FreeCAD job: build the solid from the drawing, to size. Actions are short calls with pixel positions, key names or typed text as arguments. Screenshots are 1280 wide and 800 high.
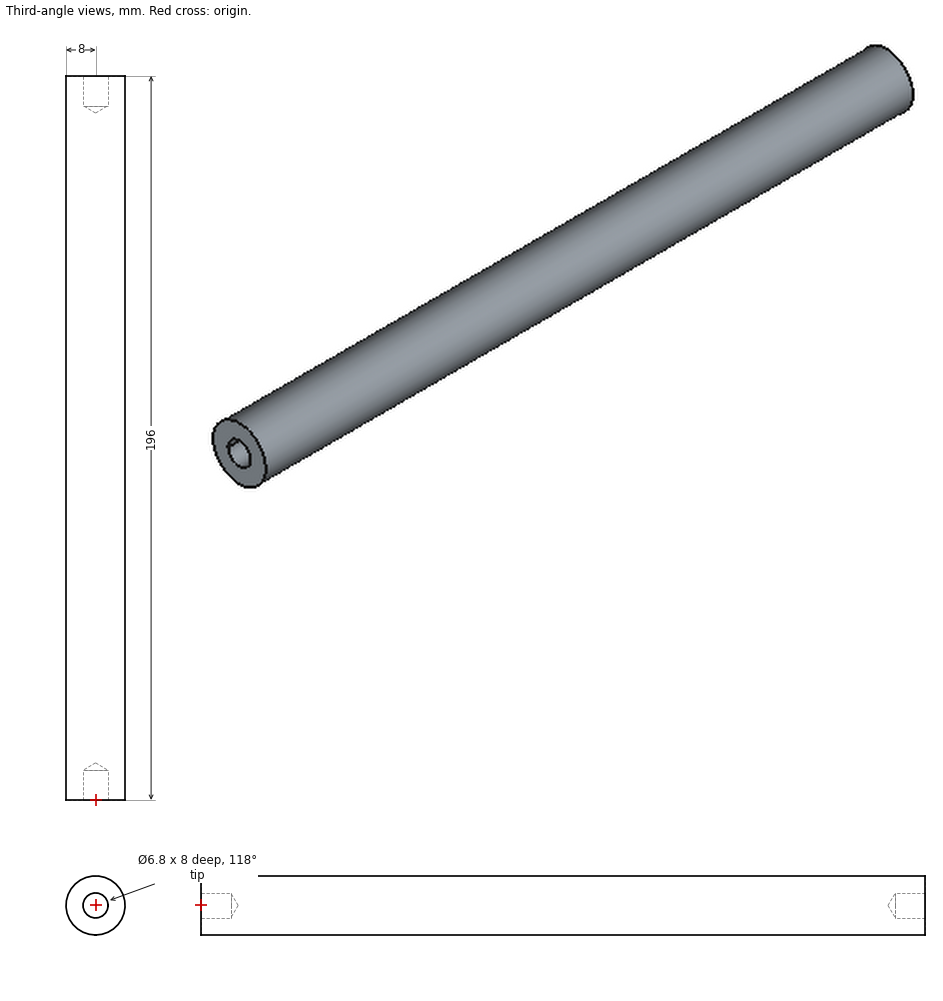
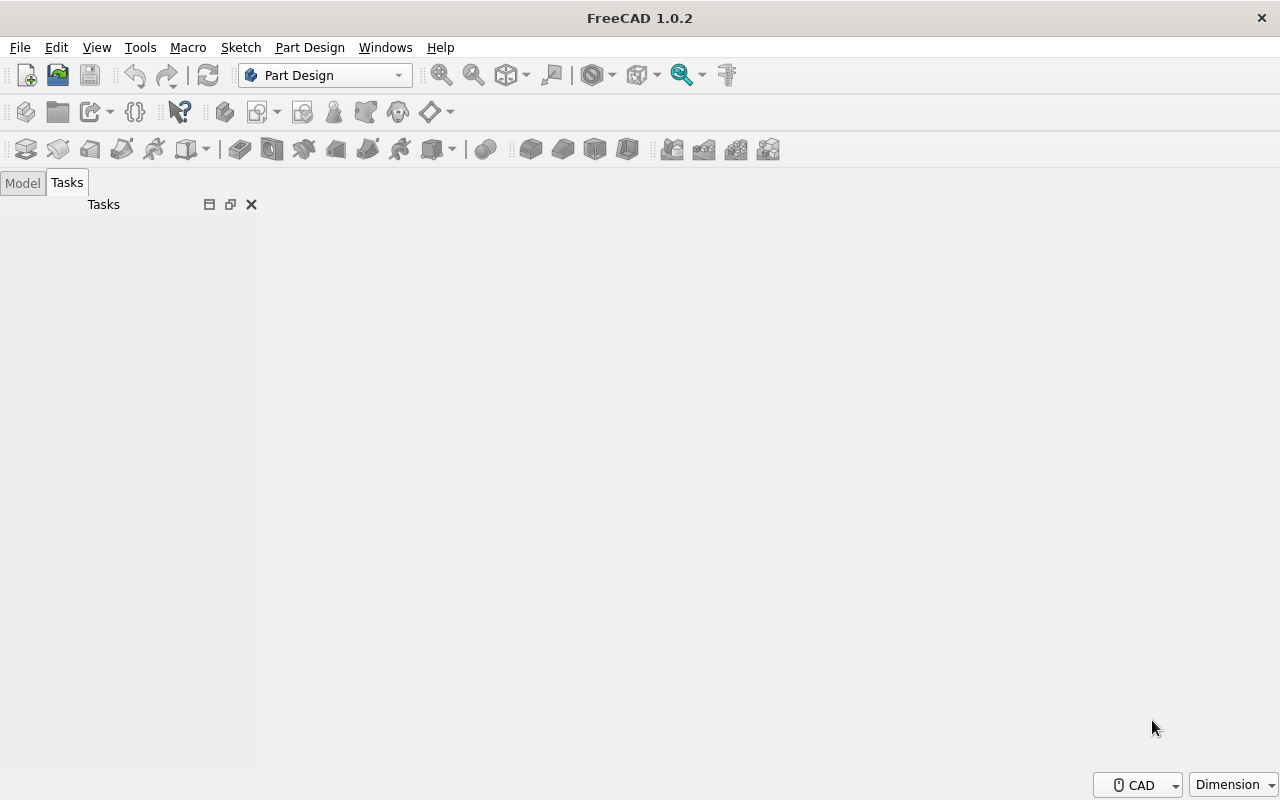
click(26, 76)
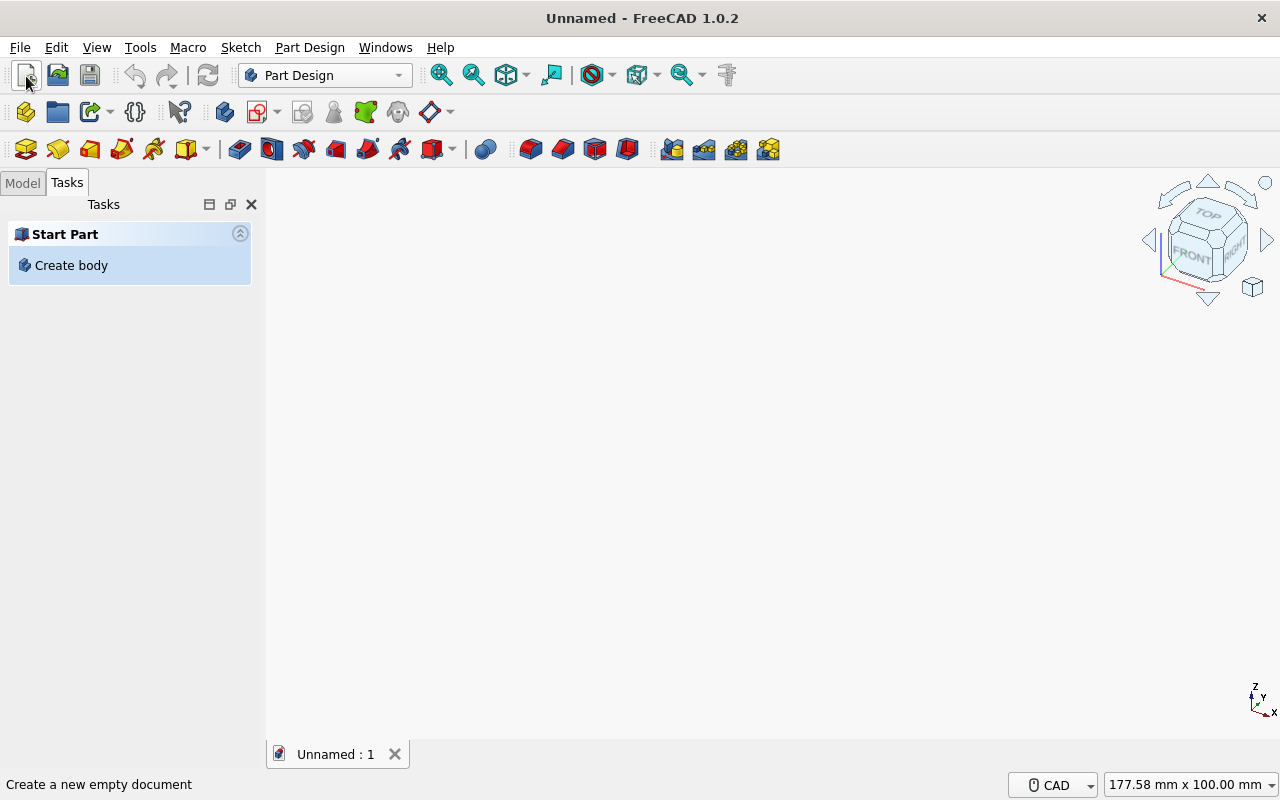
click(258, 112)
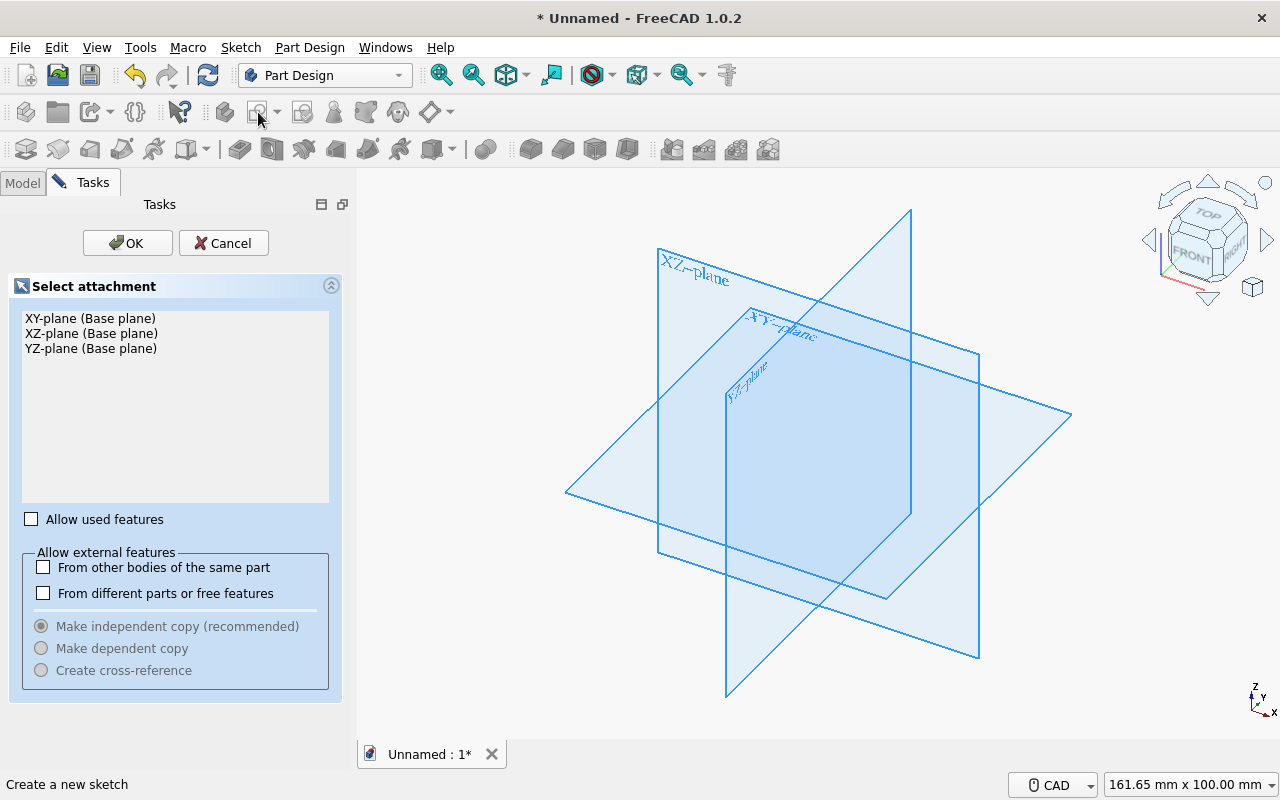
click(82, 318)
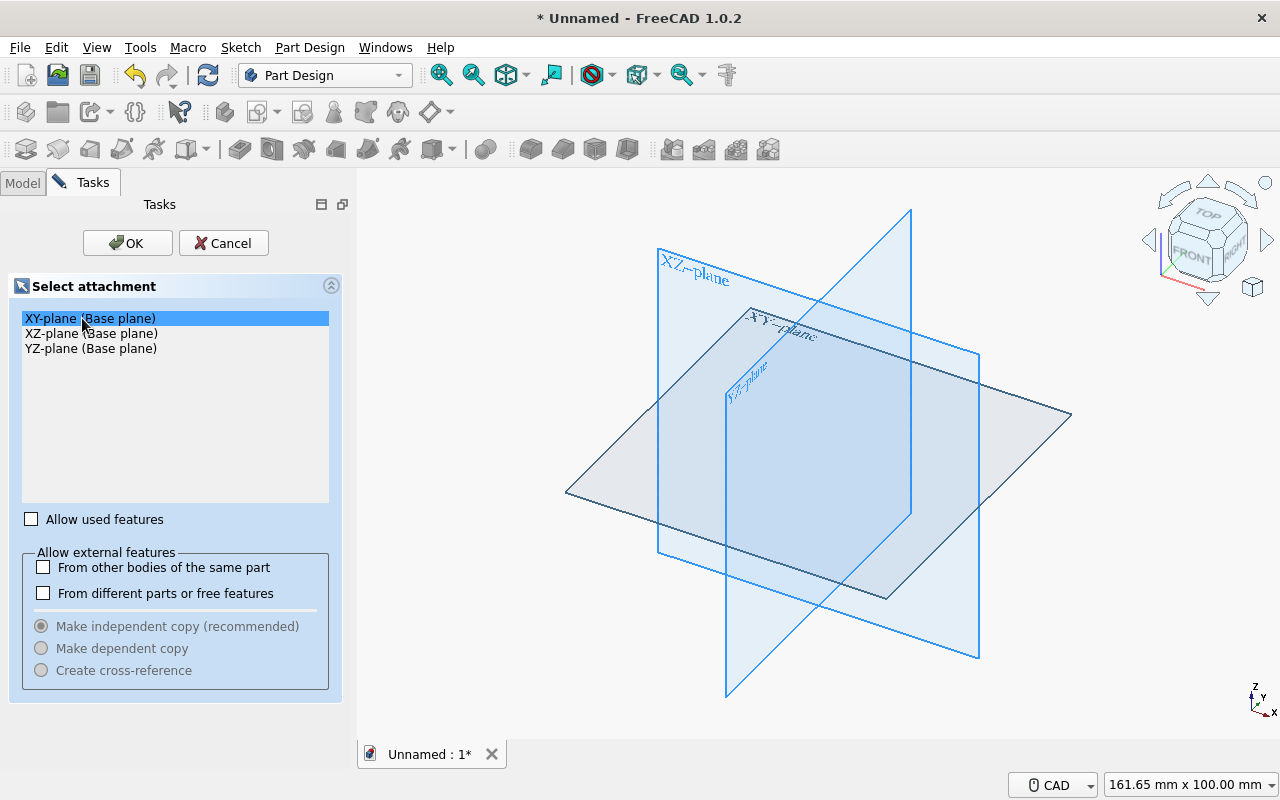
click(128, 243)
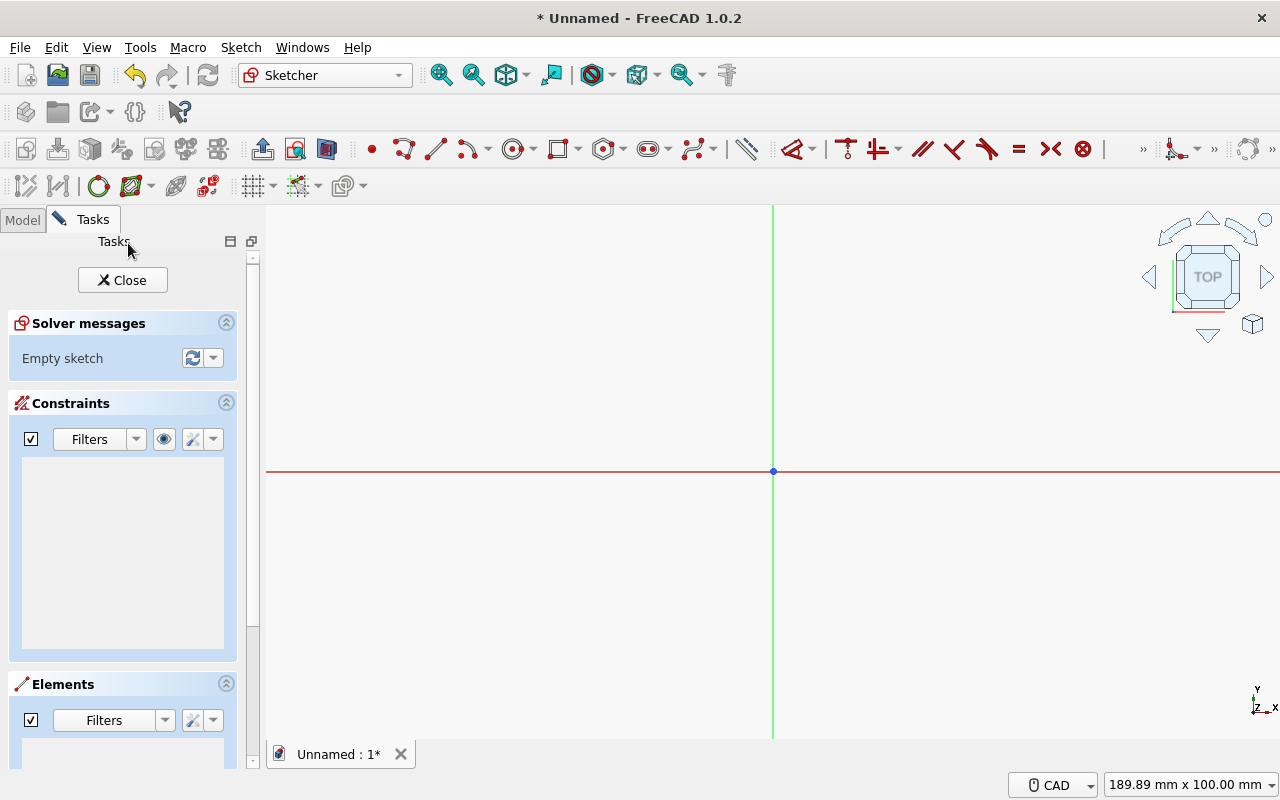
scroll(684, 698, down, 6)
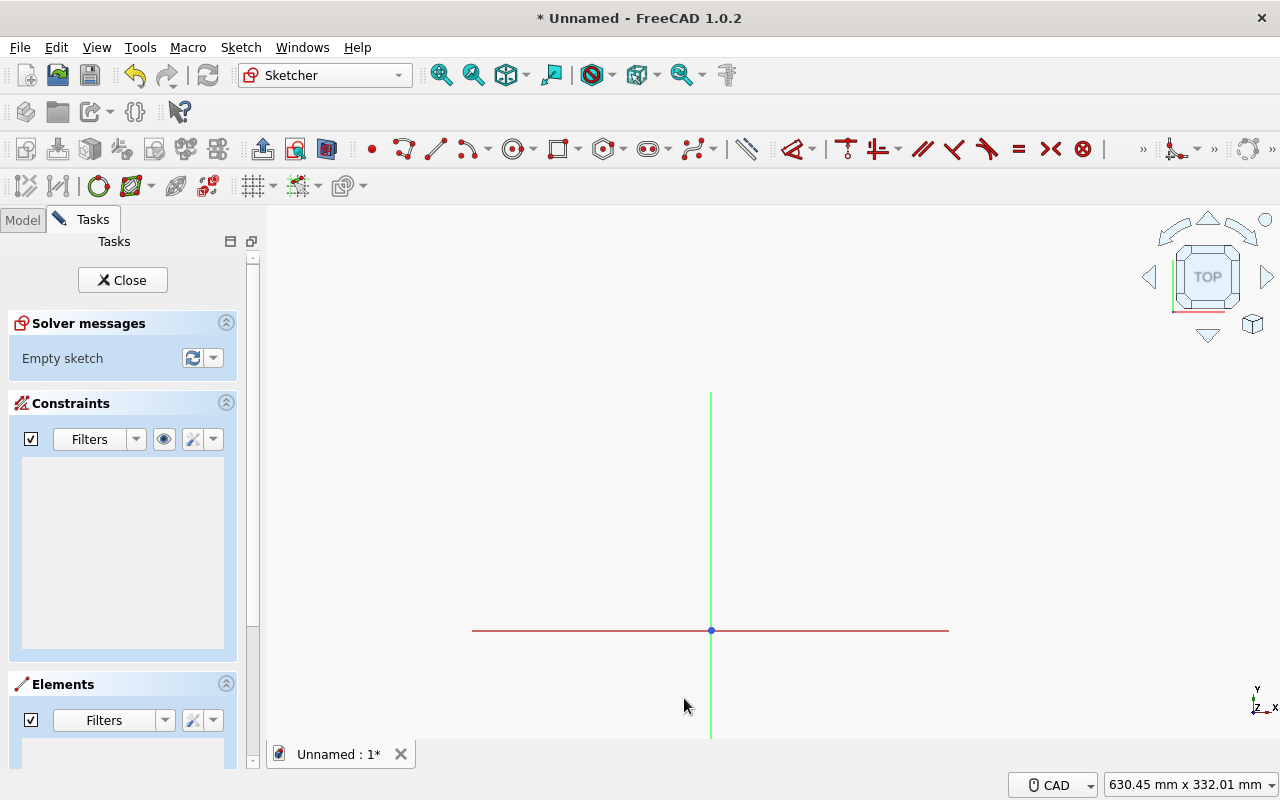
click(558, 150)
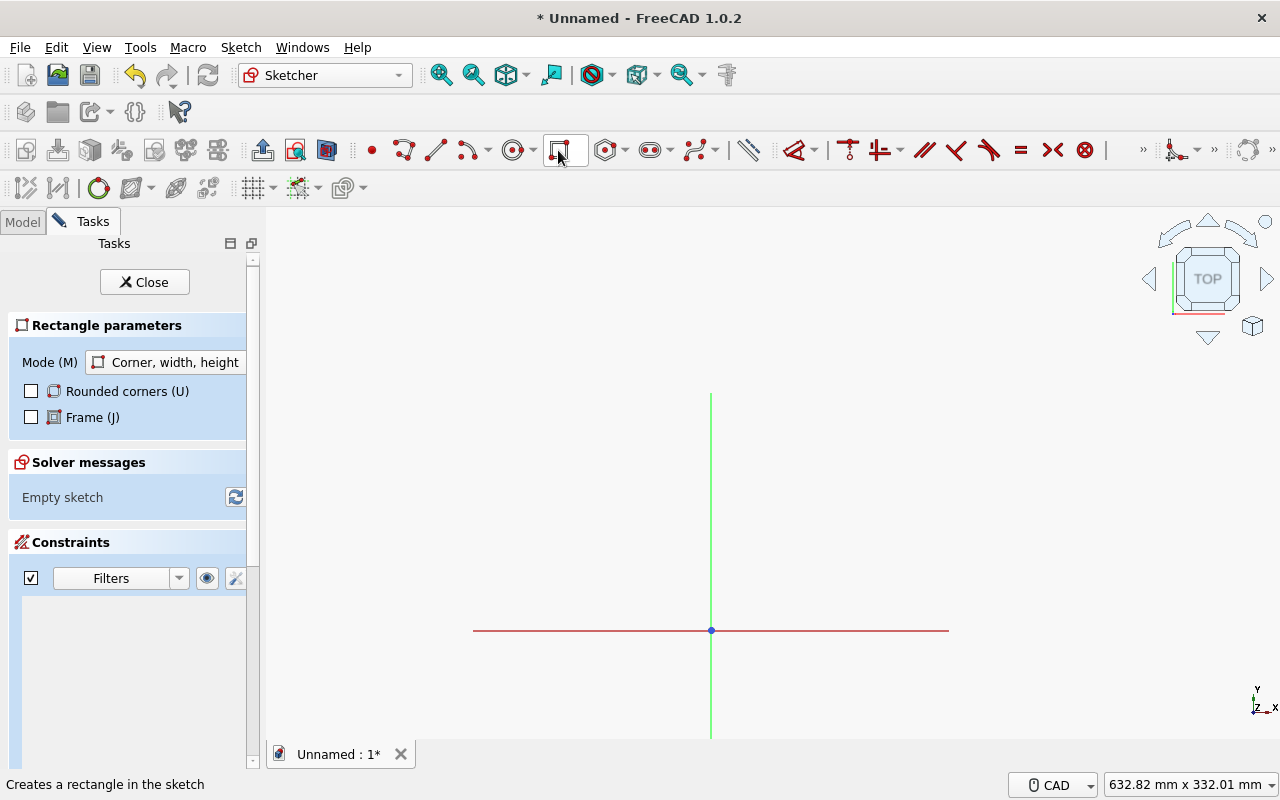
scroll(711, 631, up, 2)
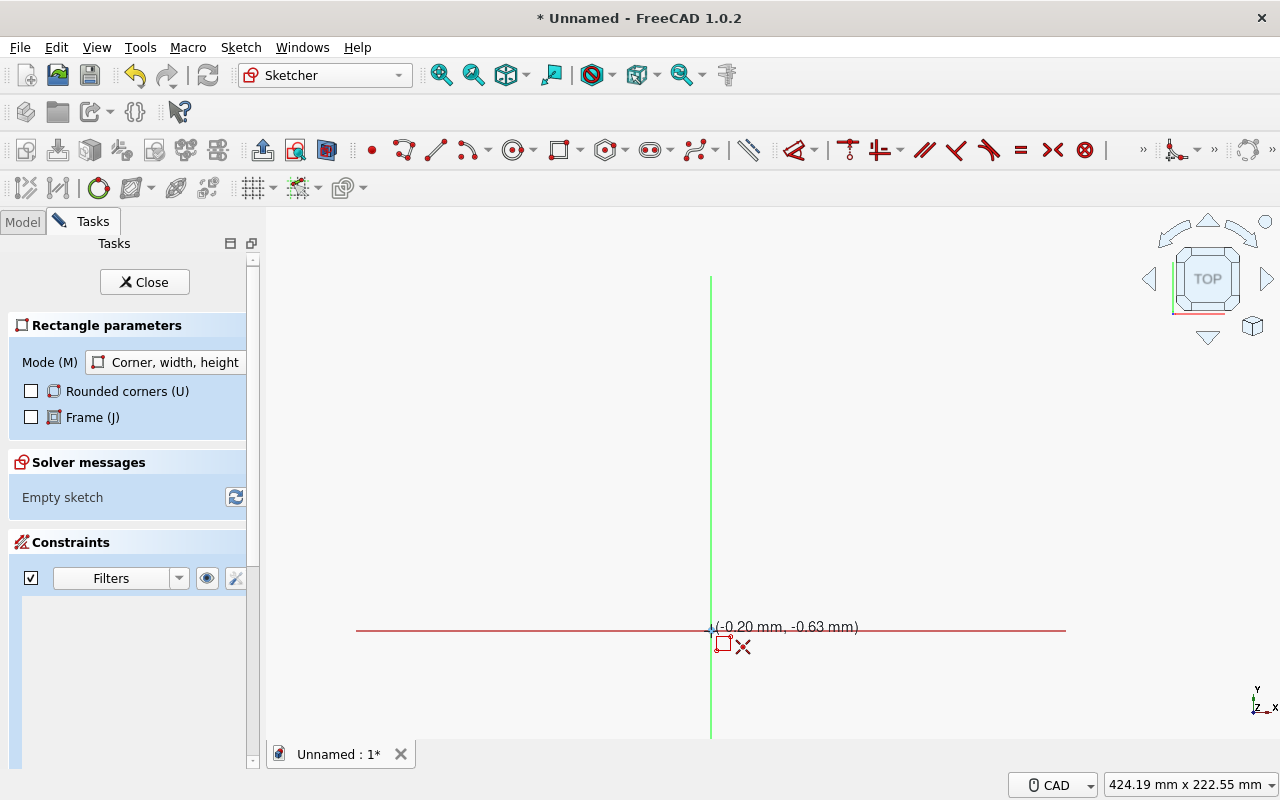
click(711, 631)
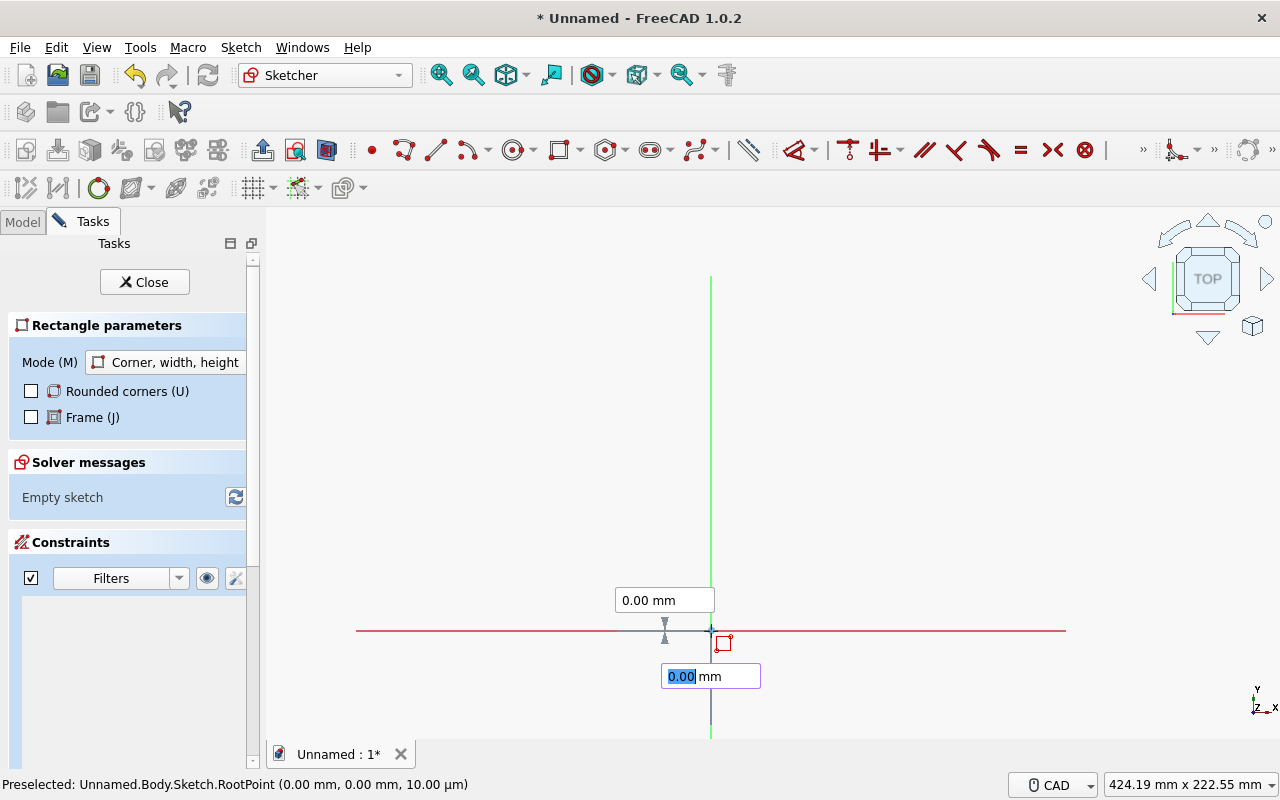
scroll(710, 629, down, 2)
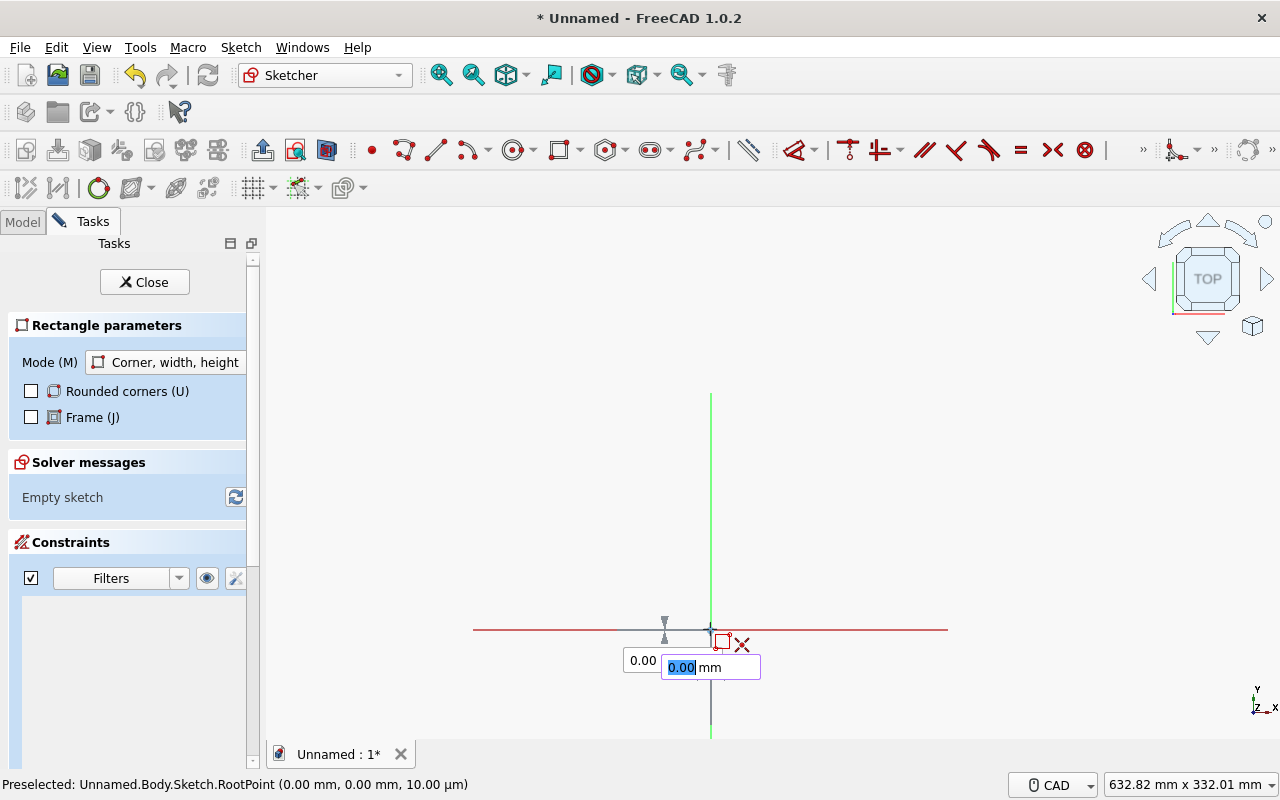
scroll(698, 316, up, 2)